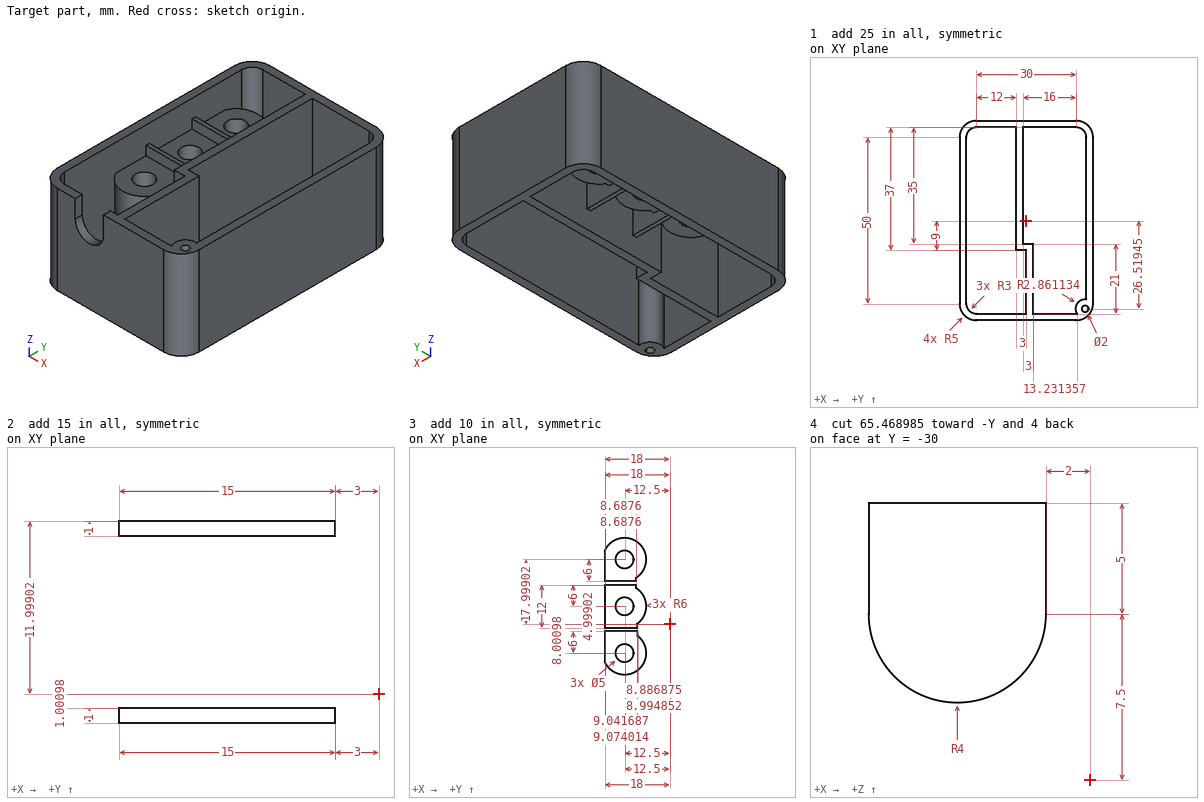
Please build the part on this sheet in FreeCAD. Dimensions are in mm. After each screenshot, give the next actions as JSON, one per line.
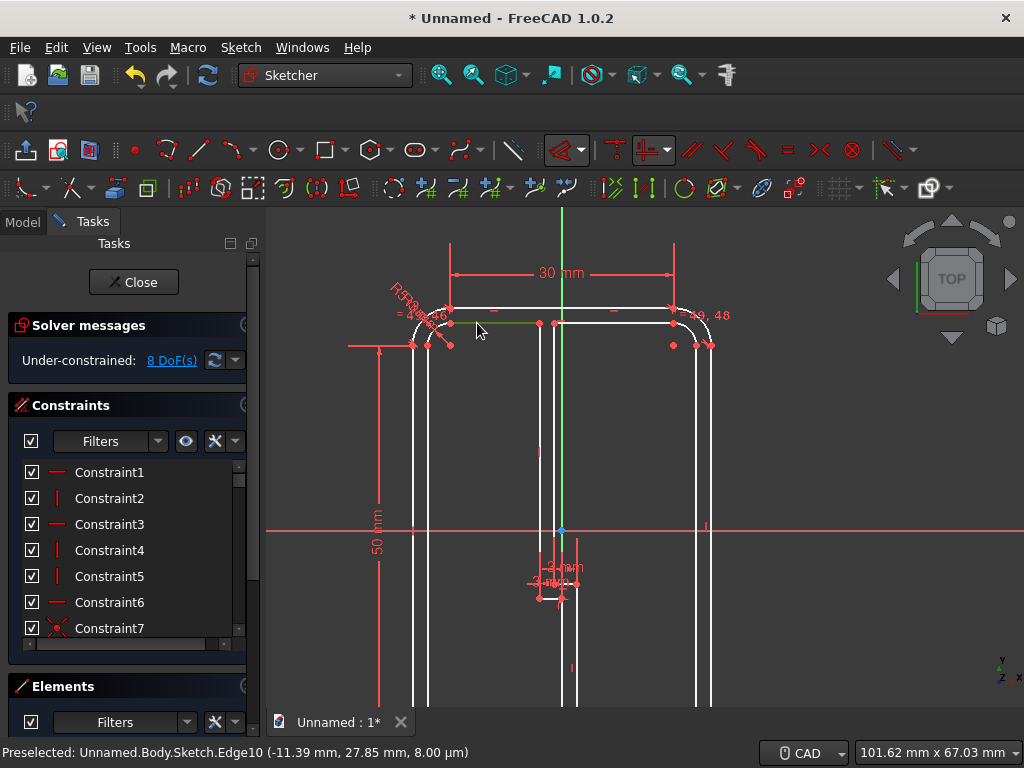
{"action": "left_click", "coordinate": [584, 150]}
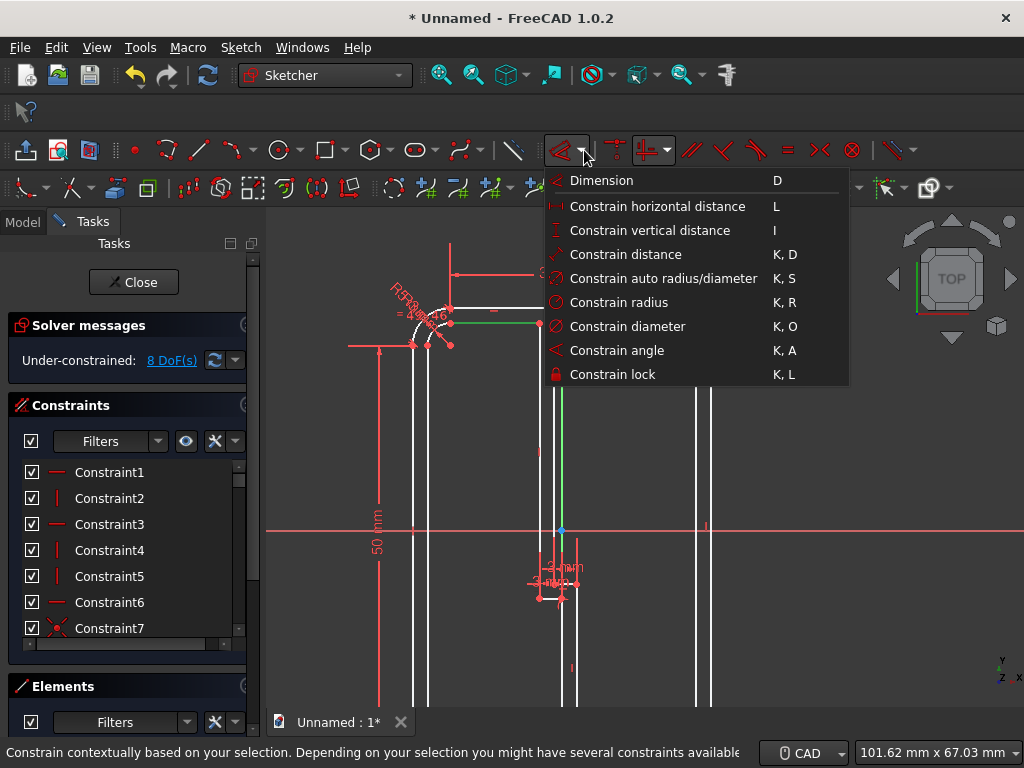
{"action": "left_click", "coordinate": [697, 206]}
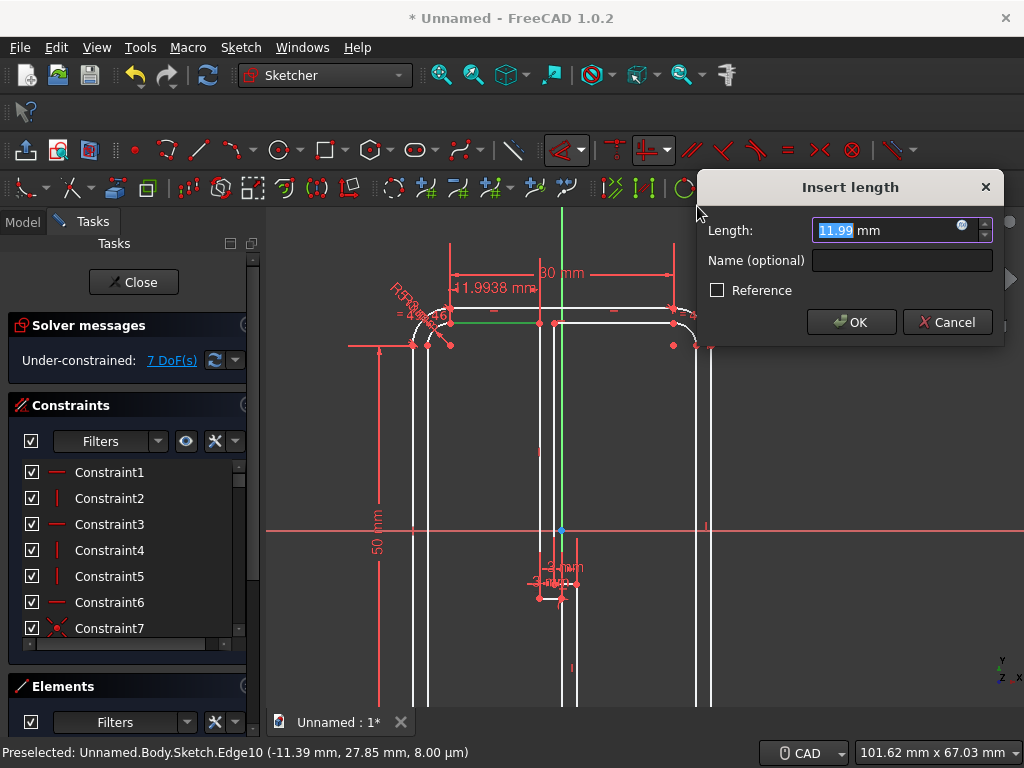
{"action": "type", "text": "12"}
{"action": "key", "text": "Return"}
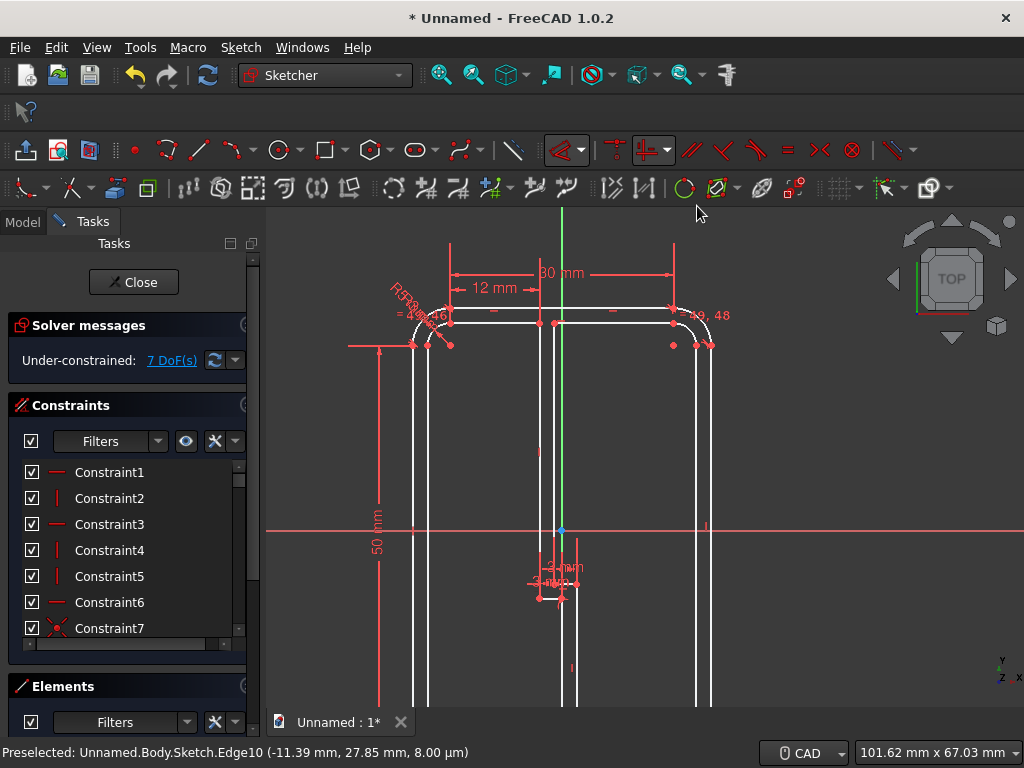
{"action": "left_click", "coordinate": [540, 406]}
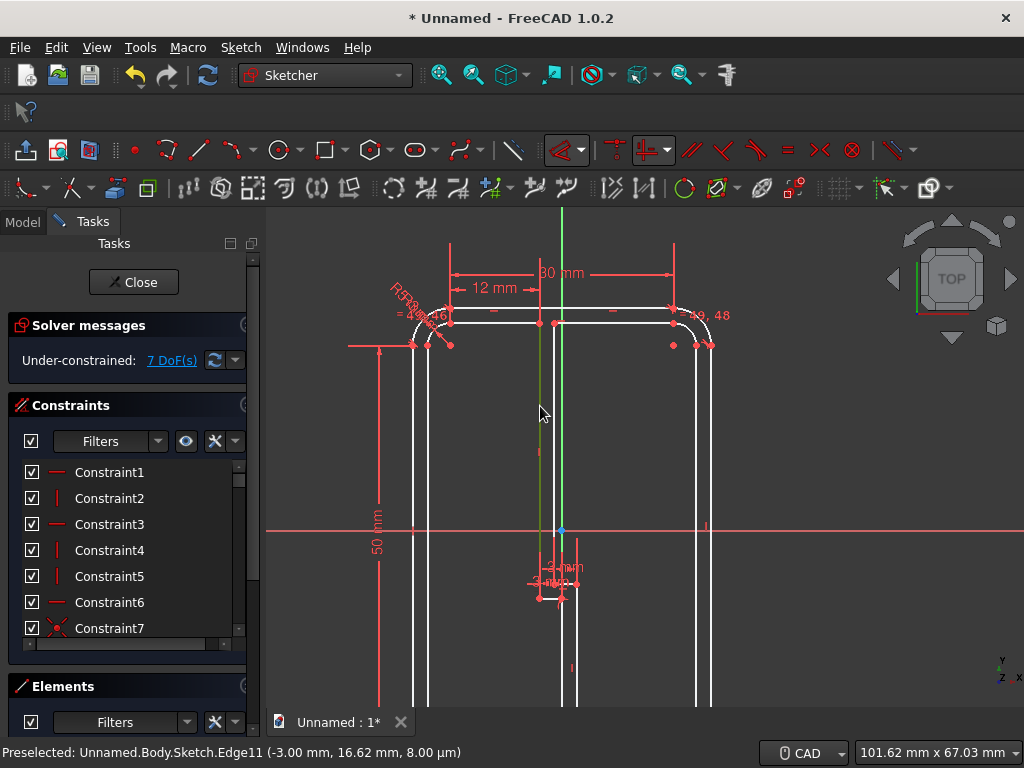
{"action": "left_click", "coordinate": [584, 150]}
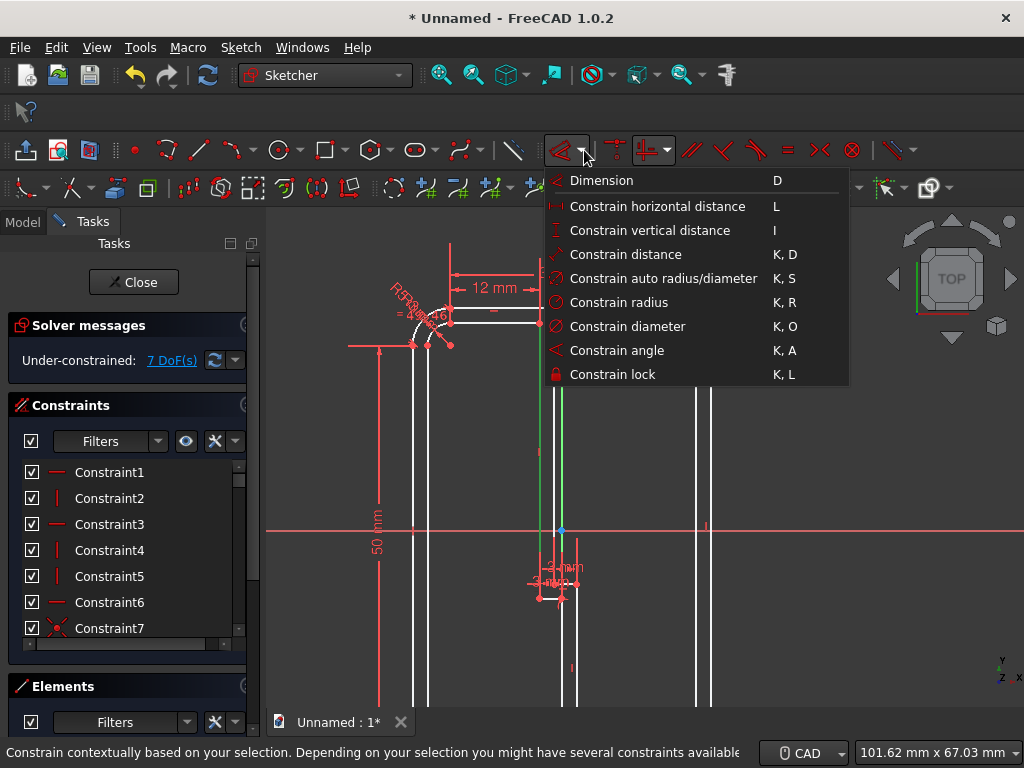
{"action": "left_click", "coordinate": [697, 230]}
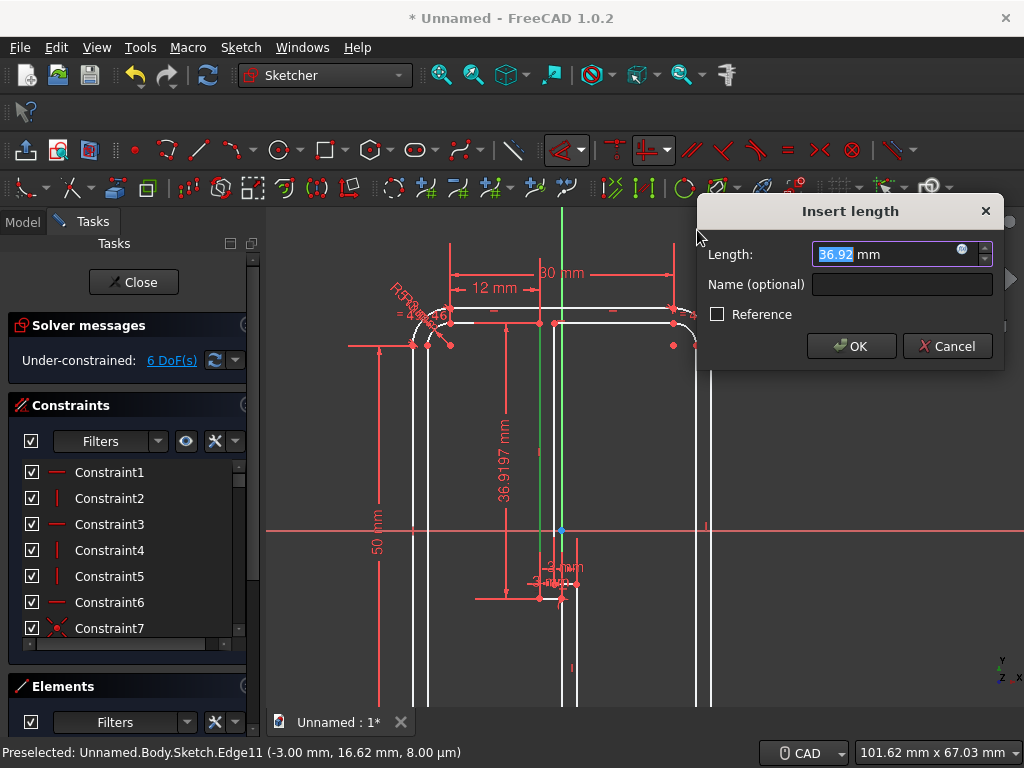
{"action": "type", "text": "37"}
{"action": "key", "text": "Return"}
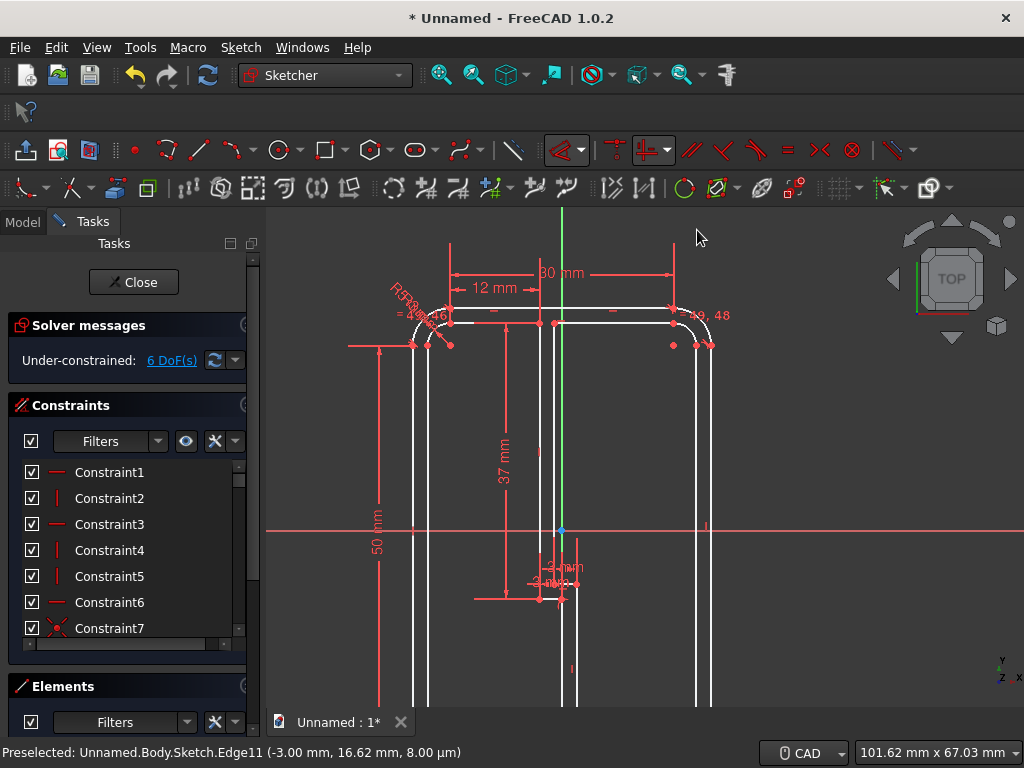
{"action": "left_click", "coordinate": [577, 631]}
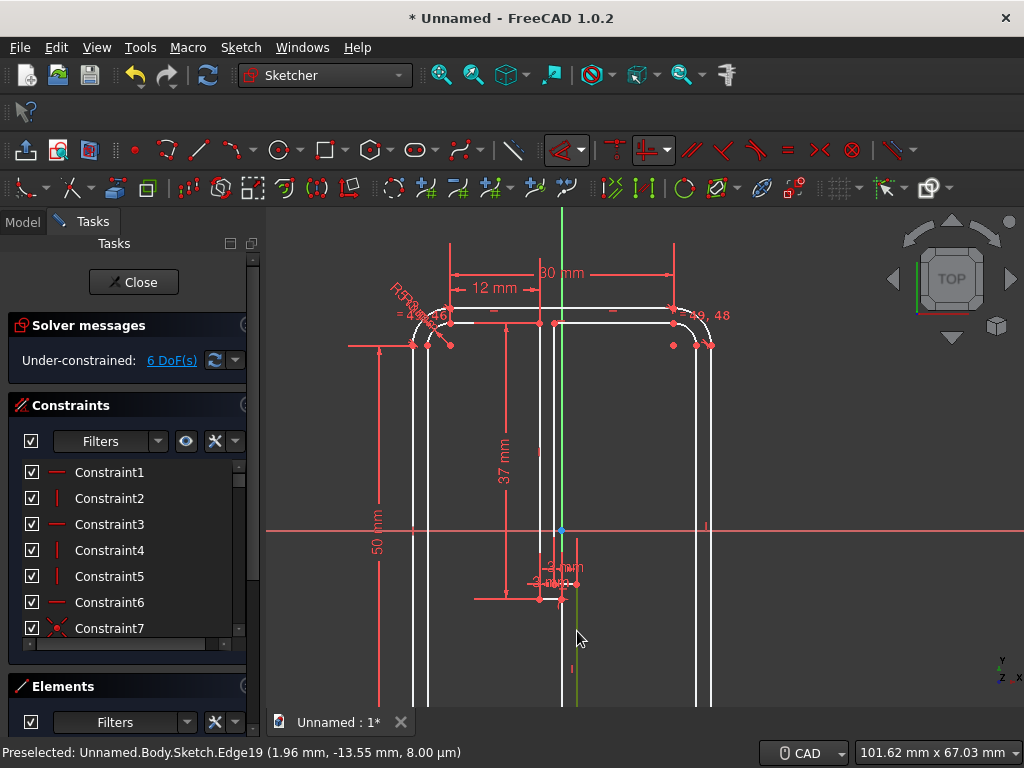
{"action": "left_click", "coordinate": [584, 150]}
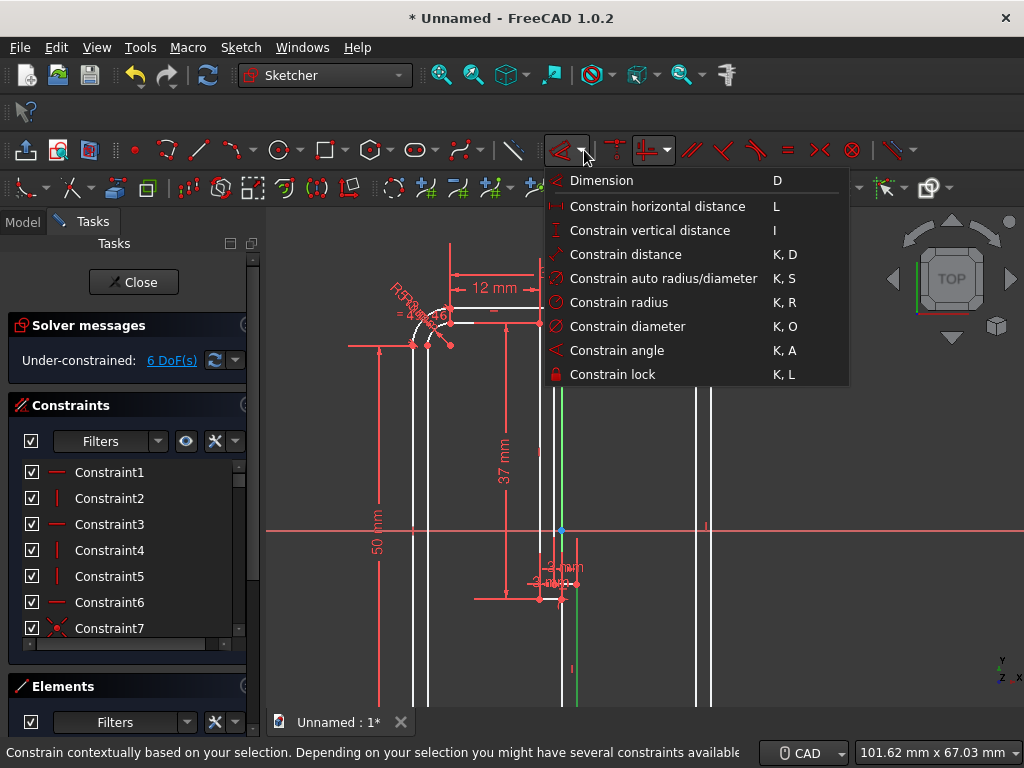
{"action": "left_click", "coordinate": [697, 230]}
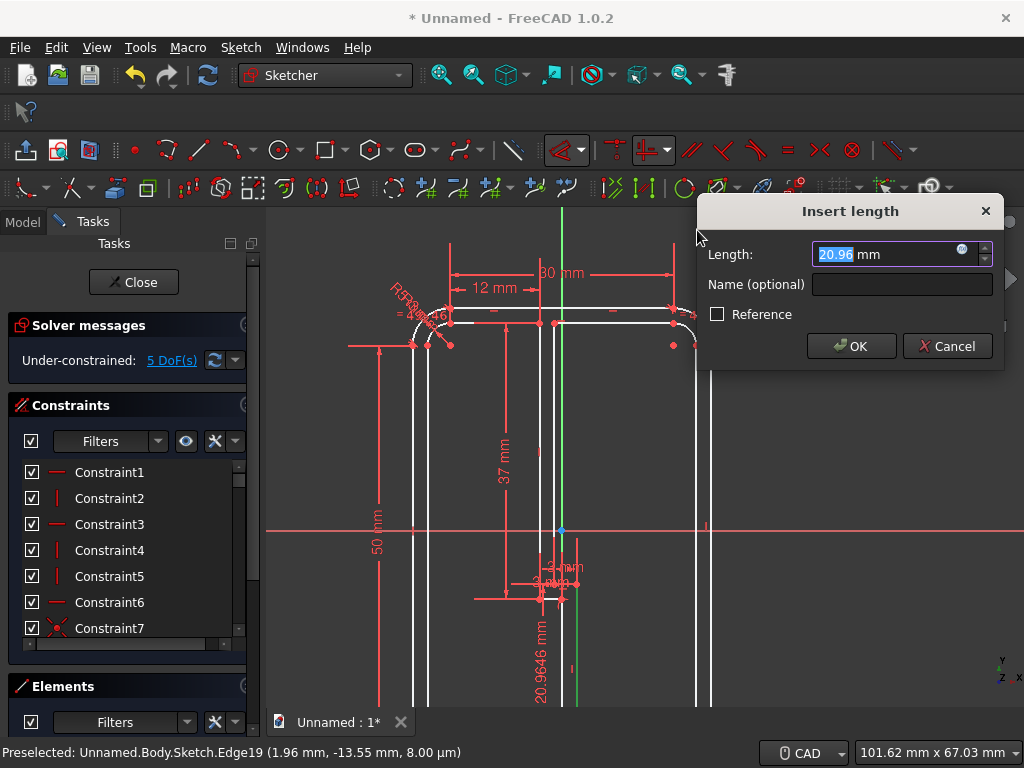
{"action": "type", "text": "21"}
{"action": "key", "text": "Return"}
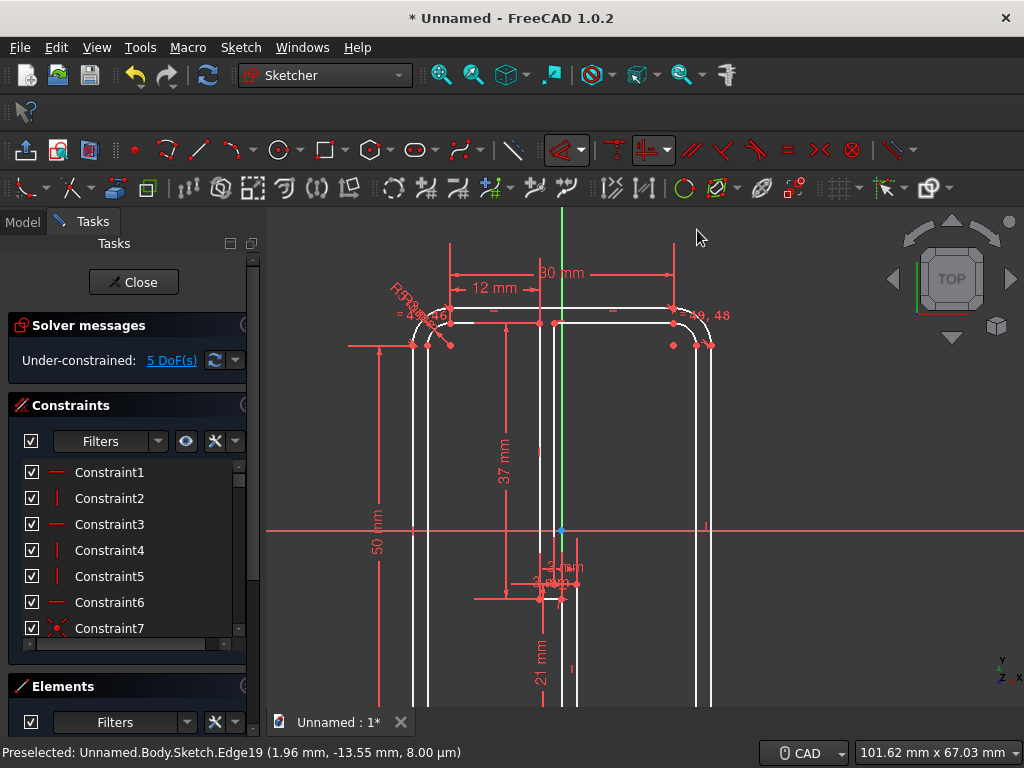
{"action": "scroll", "coordinate": [554, 506], "scroll_direction": "up", "scroll_amount": 3}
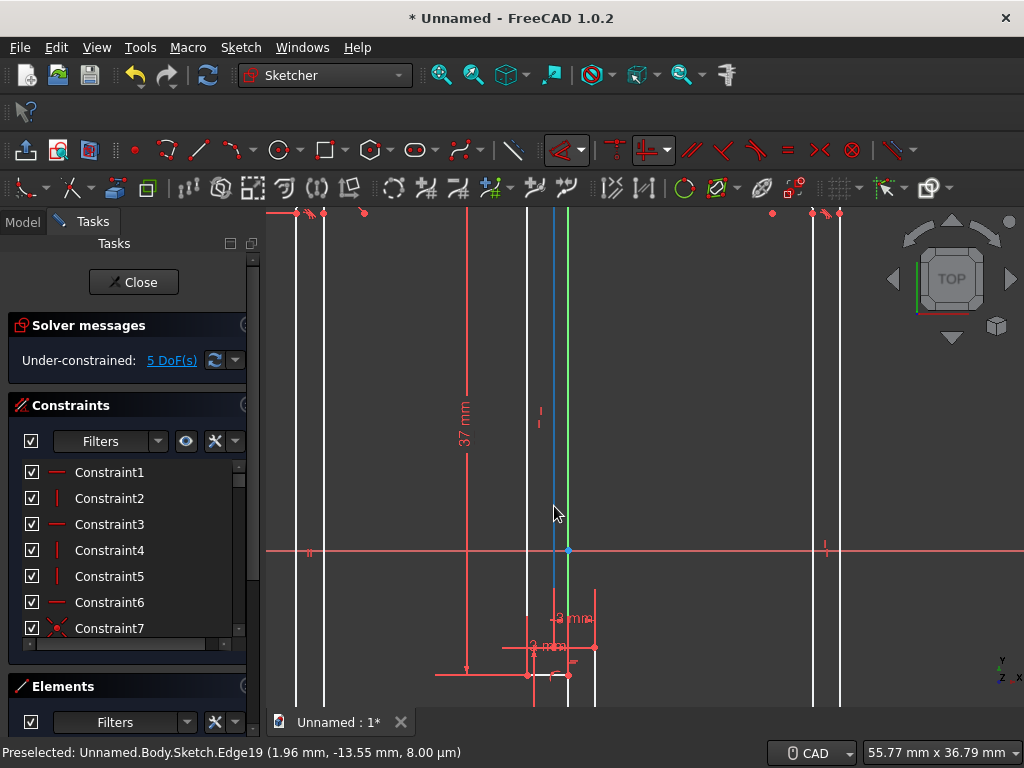
{"action": "left_click", "coordinate": [554, 505]}